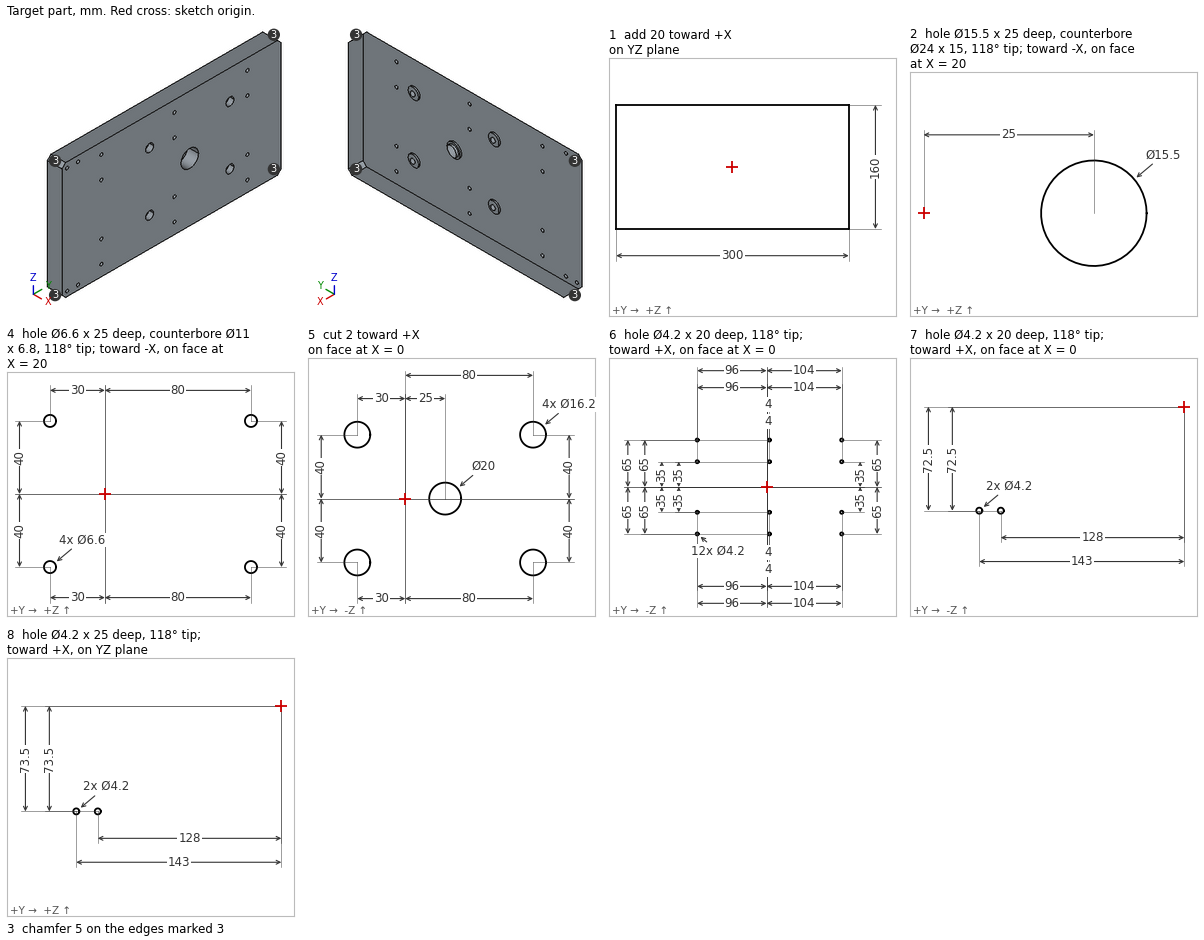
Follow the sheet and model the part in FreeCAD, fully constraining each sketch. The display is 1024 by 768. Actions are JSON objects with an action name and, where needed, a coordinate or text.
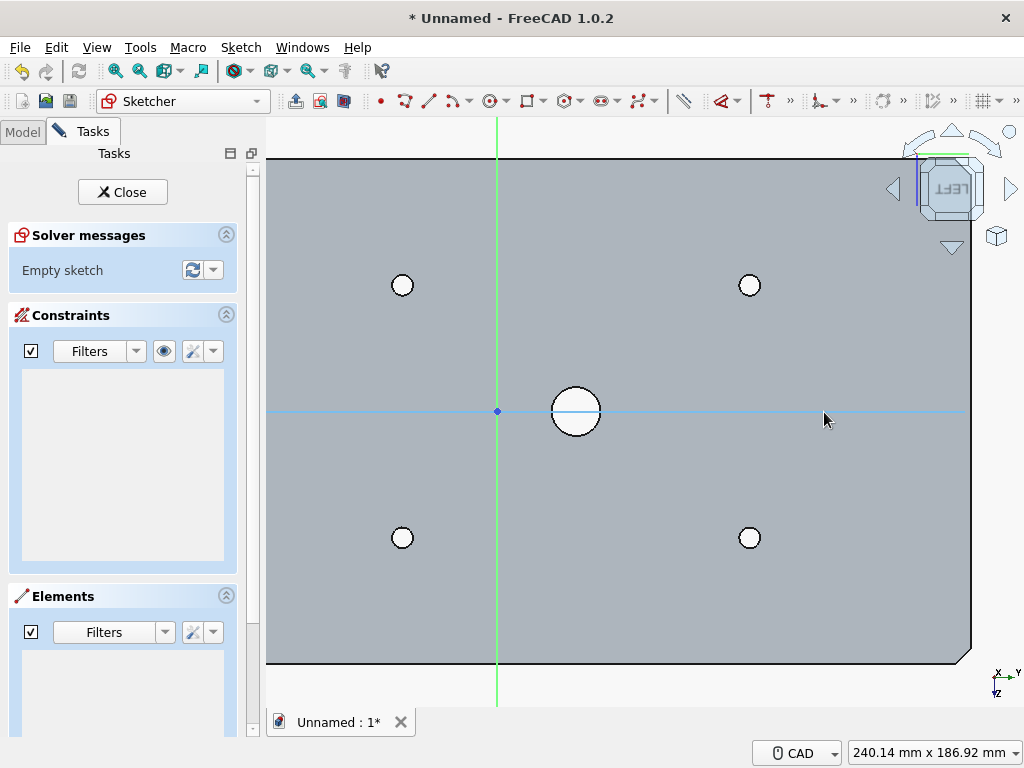
{"action": "key", "text": "g c"}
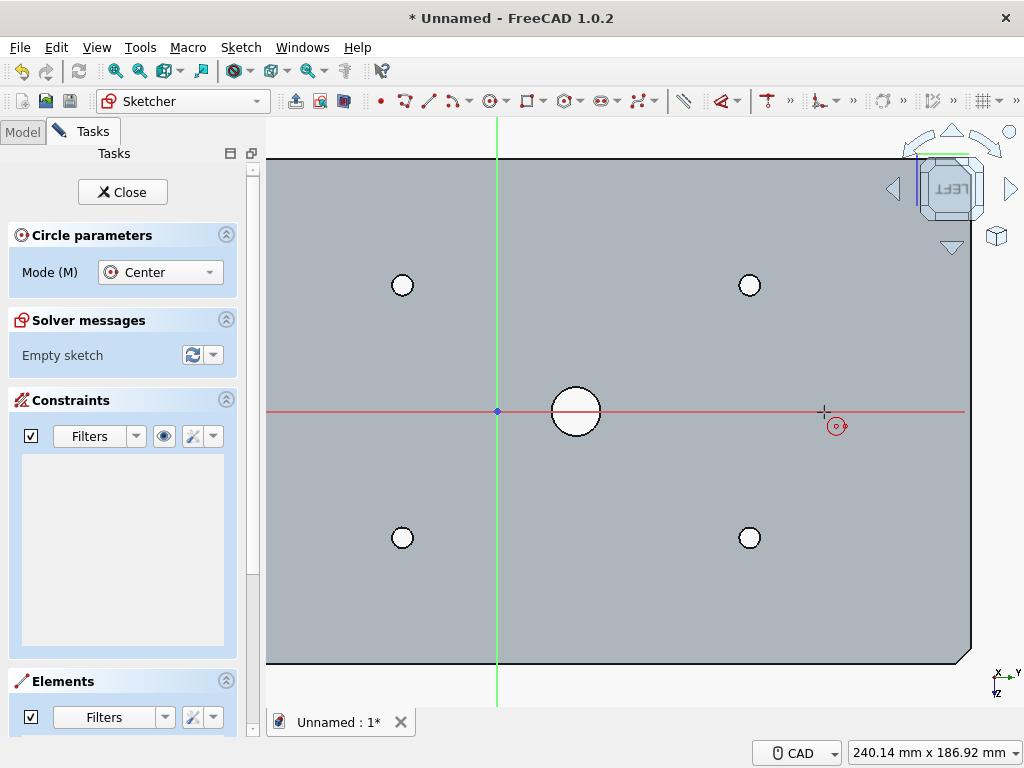
{"action": "left_click", "coordinate": [750, 285]}
{"action": "left_click", "coordinate": [768, 267]}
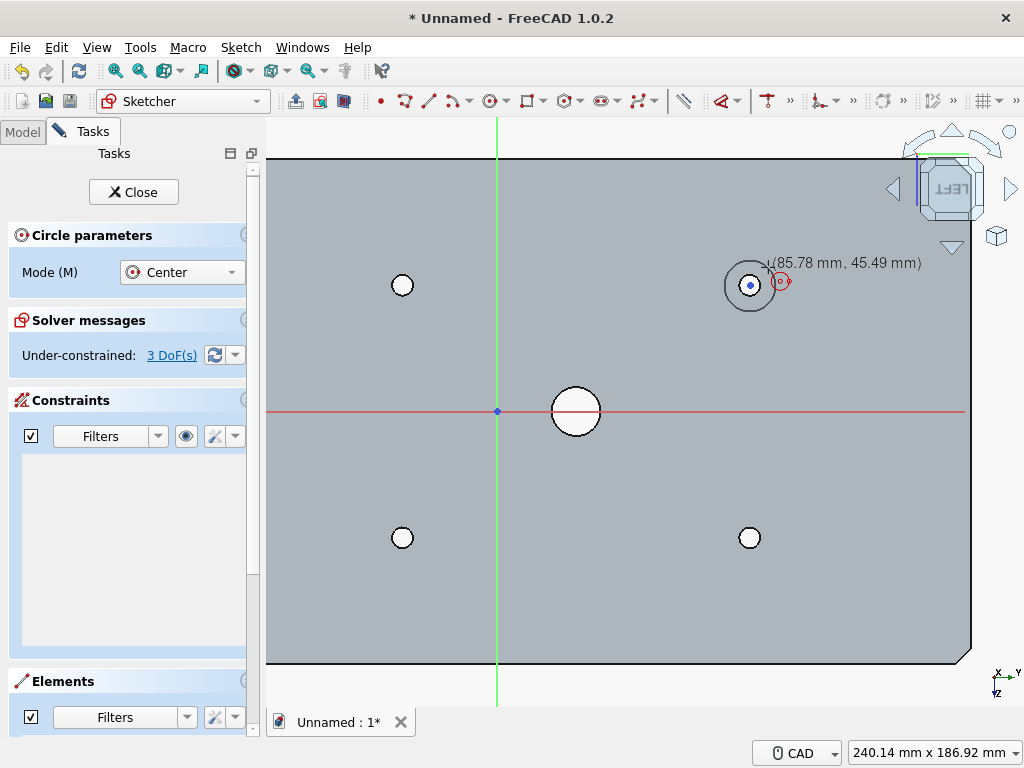
{"action": "left_click", "coordinate": [403, 285]}
{"action": "left_click", "coordinate": [421, 267]}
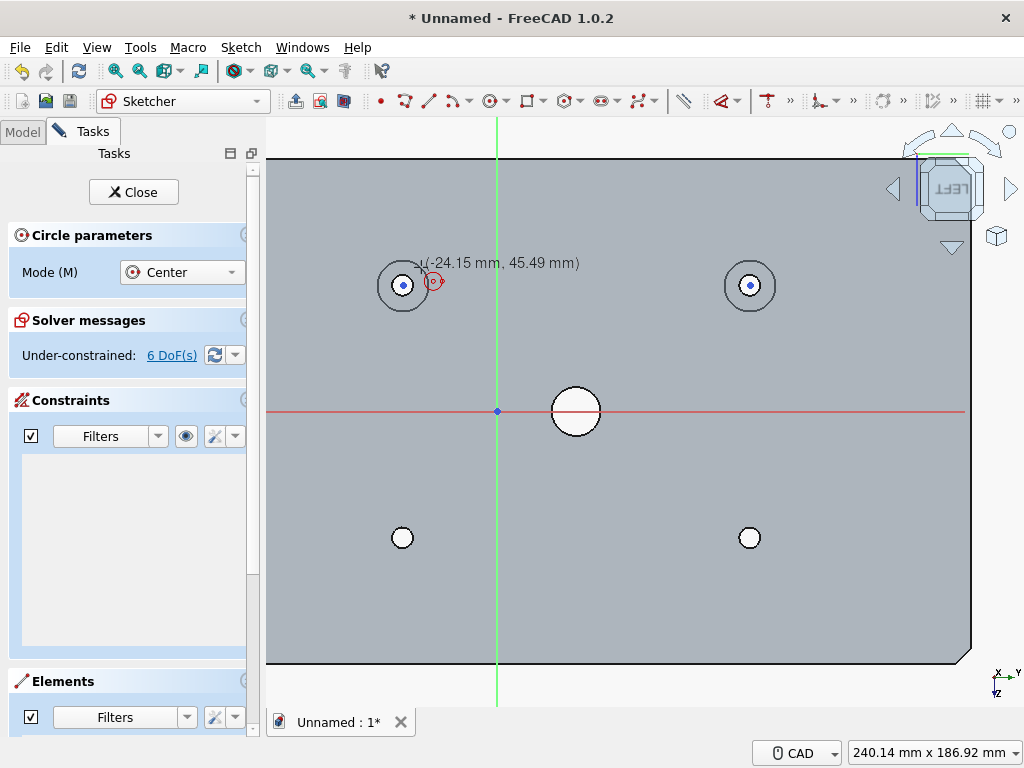
{"action": "left_click", "coordinate": [576, 412]}
{"action": "left_click", "coordinate": [598, 389]}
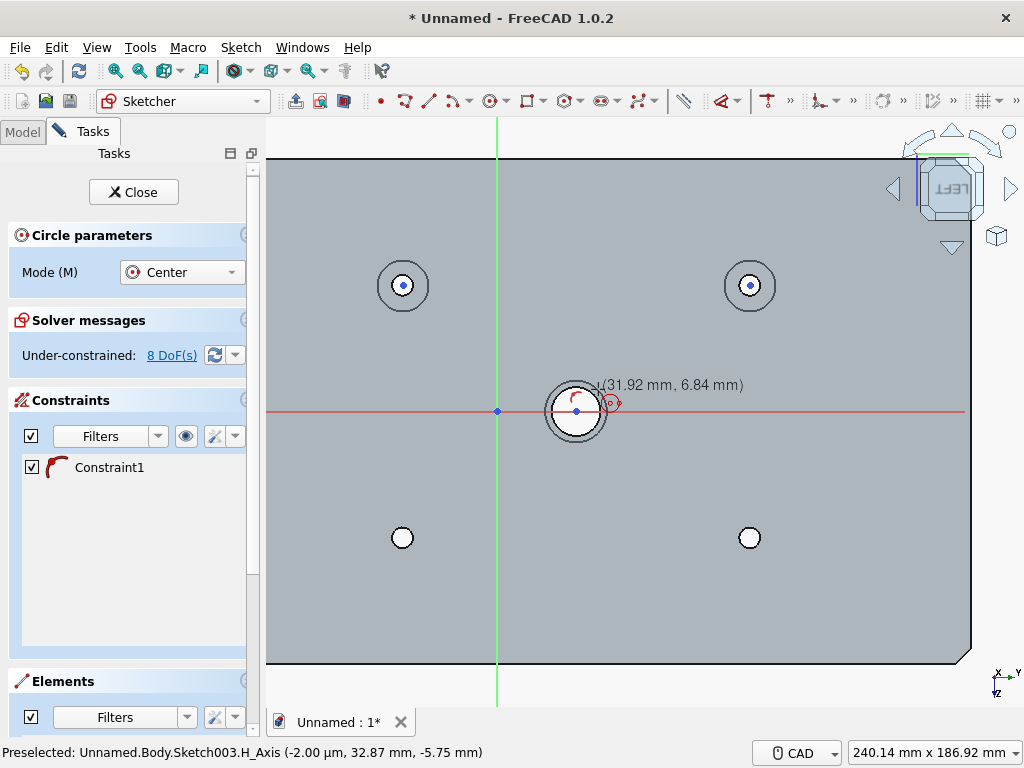
{"action": "left_click", "coordinate": [403, 538]}
{"action": "left_click", "coordinate": [421, 520]}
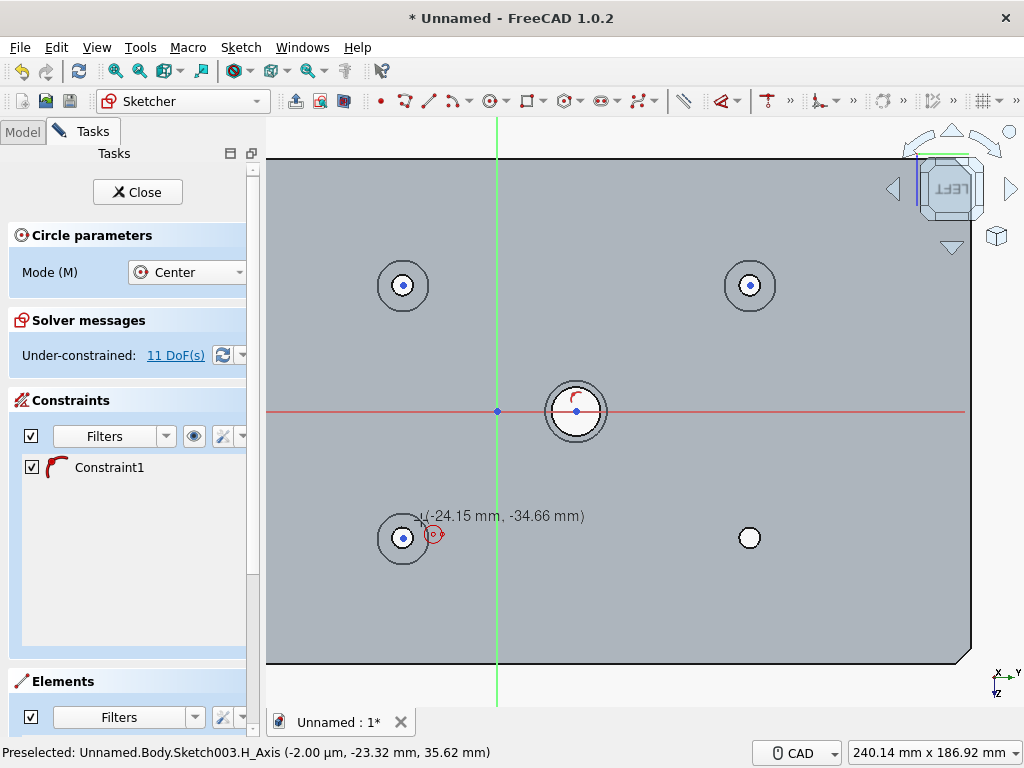
{"action": "left_click", "coordinate": [750, 538]}
{"action": "left_click", "coordinate": [768, 520]}
{"action": "key", "text": "Escape"}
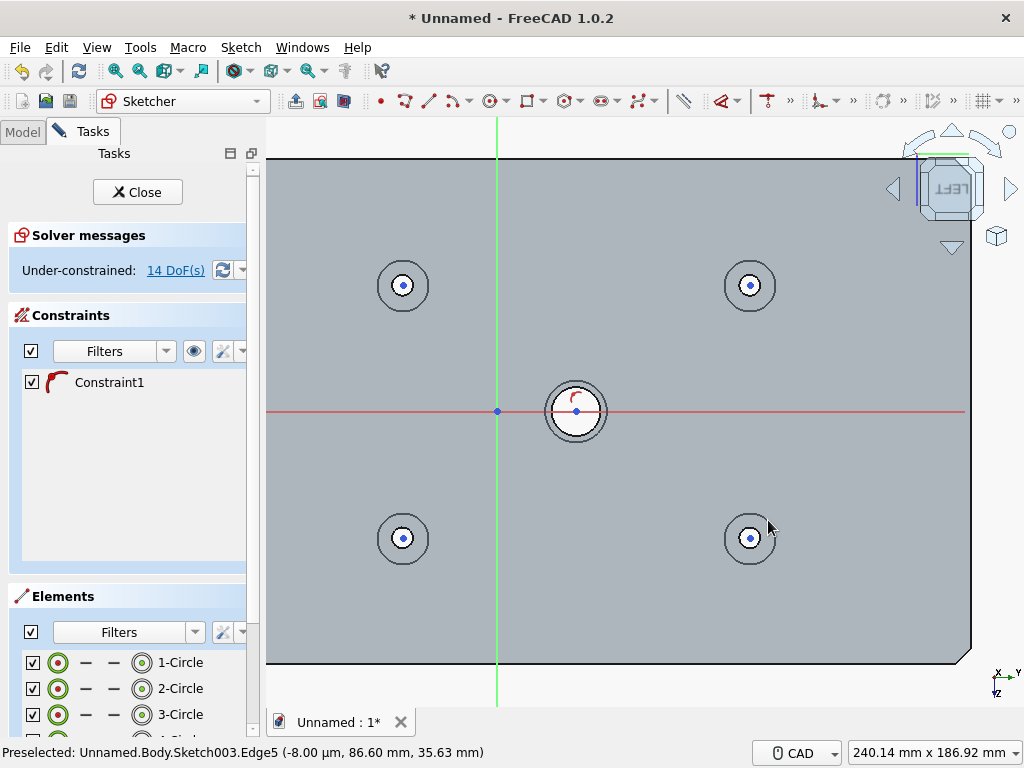
{"action": "left_click", "coordinate": [768, 268]}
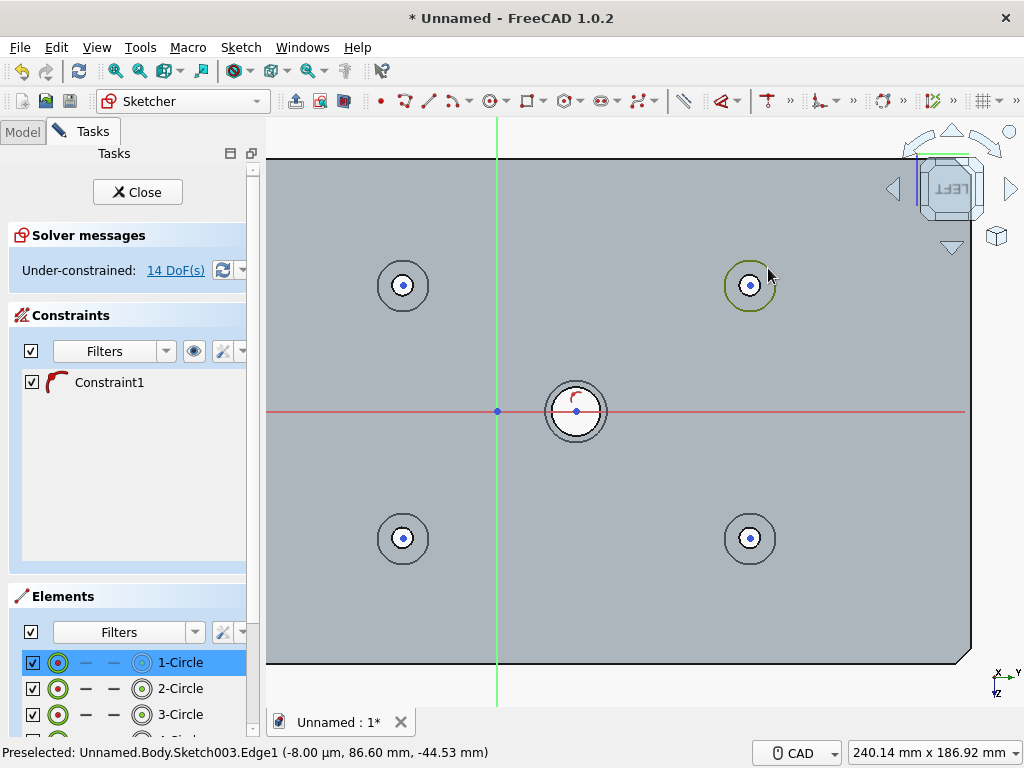
{"action": "left_click", "coordinate": [421, 268]}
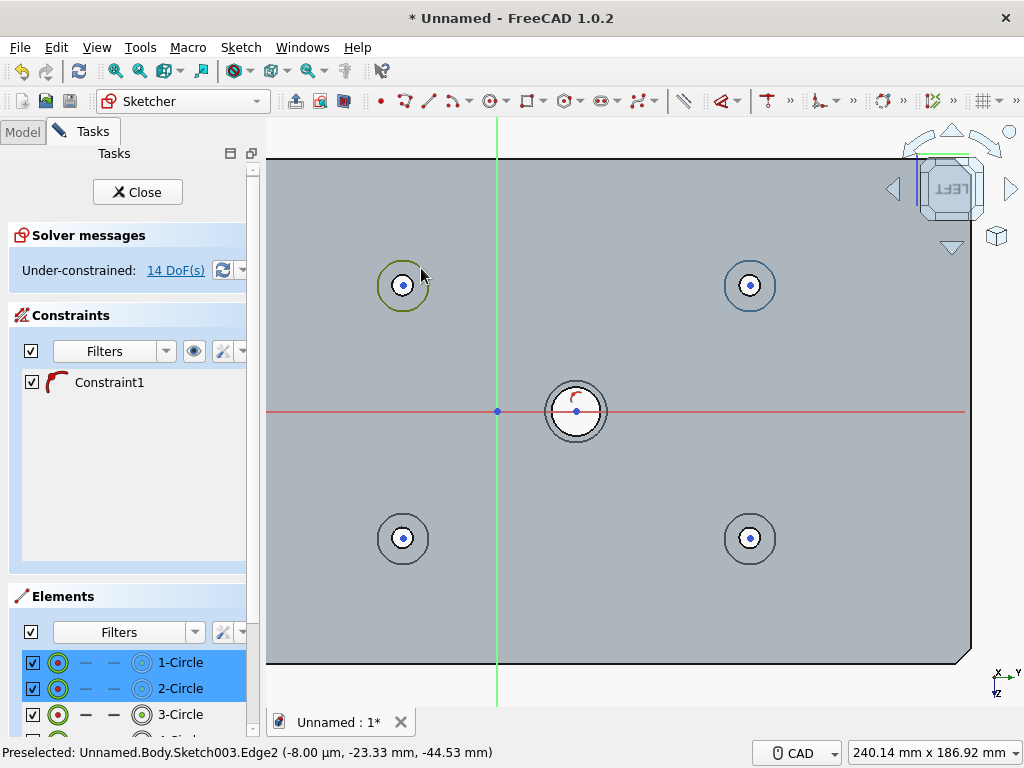
{"action": "left_click", "coordinate": [421, 521]}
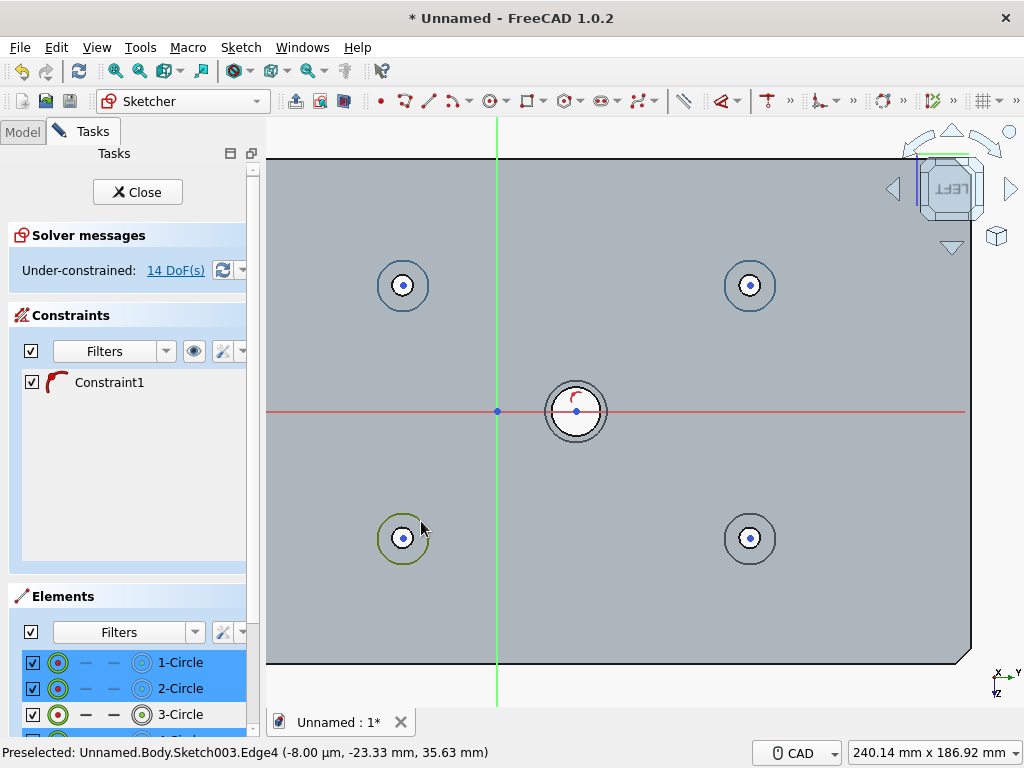
{"action": "left_click", "coordinate": [768, 521]}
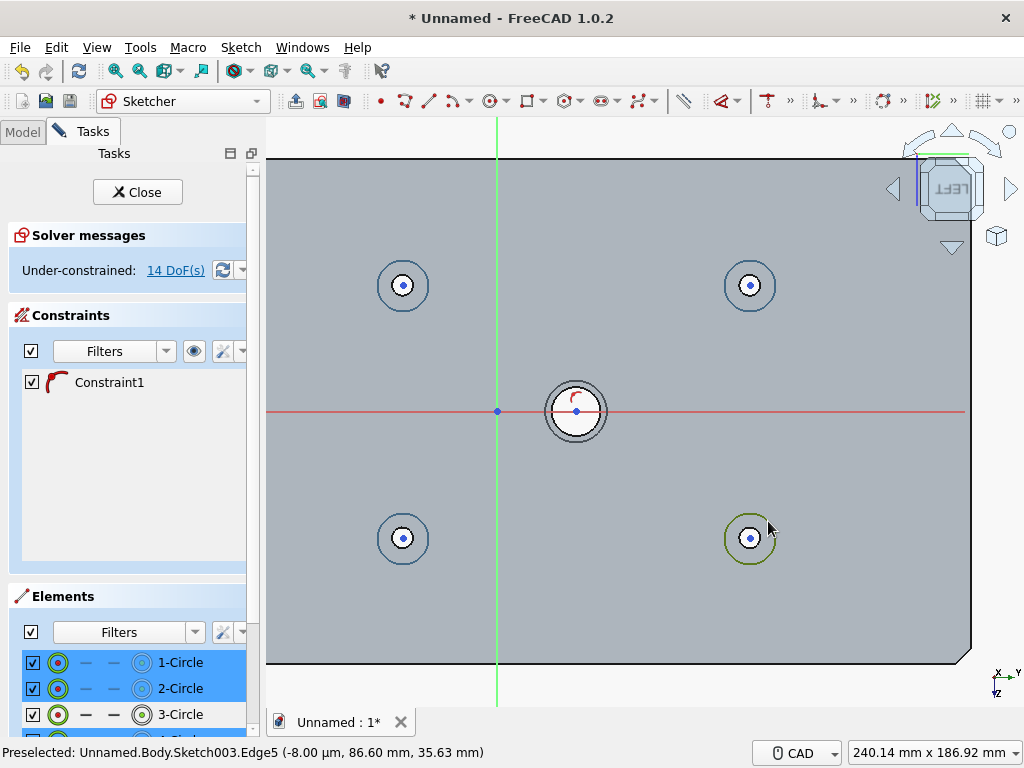
{"action": "key", "text": "e"}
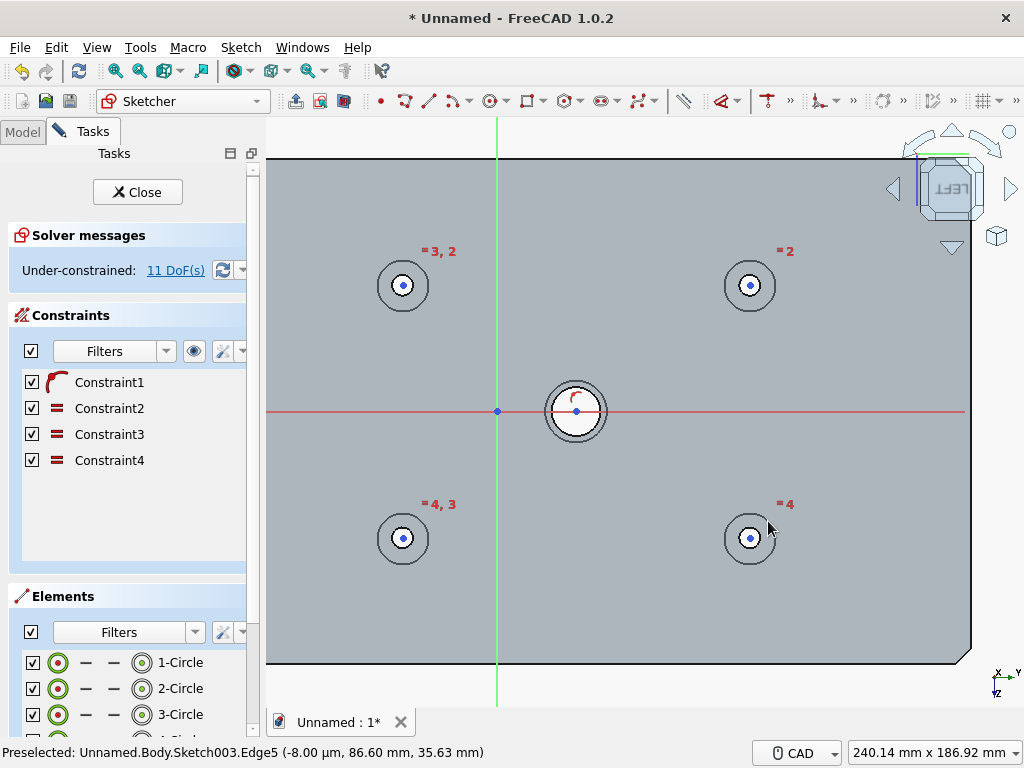
{"action": "left_click", "coordinate": [722, 102]}